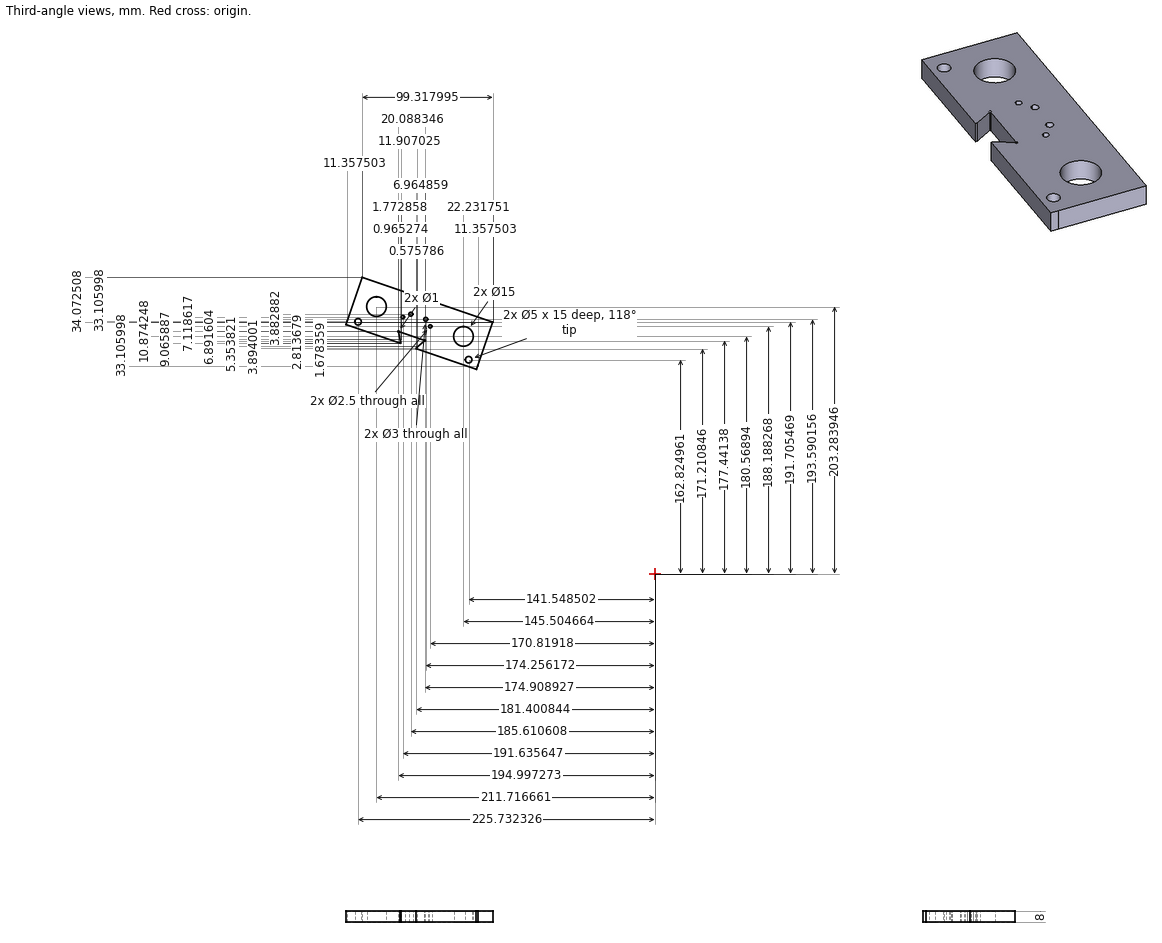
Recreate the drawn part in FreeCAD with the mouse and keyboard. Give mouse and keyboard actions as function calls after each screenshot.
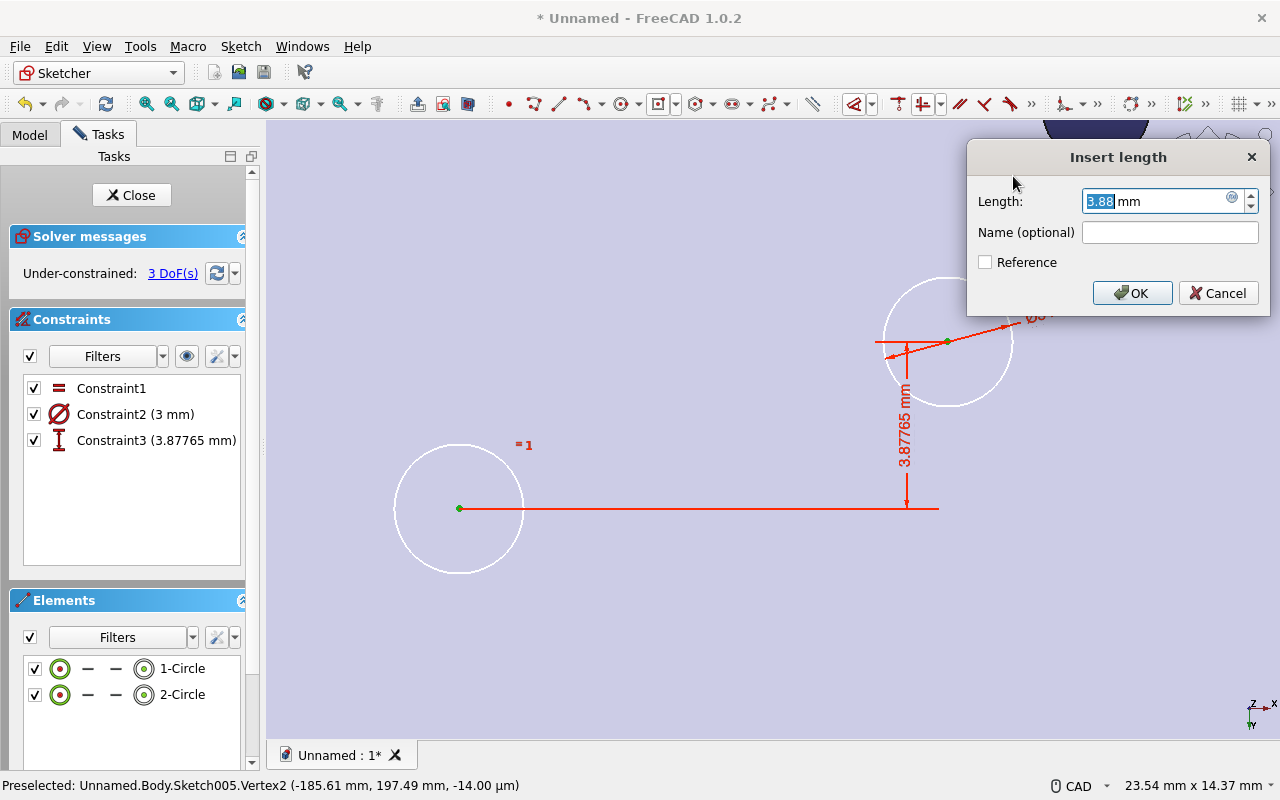
text(3.882882)
key(Return)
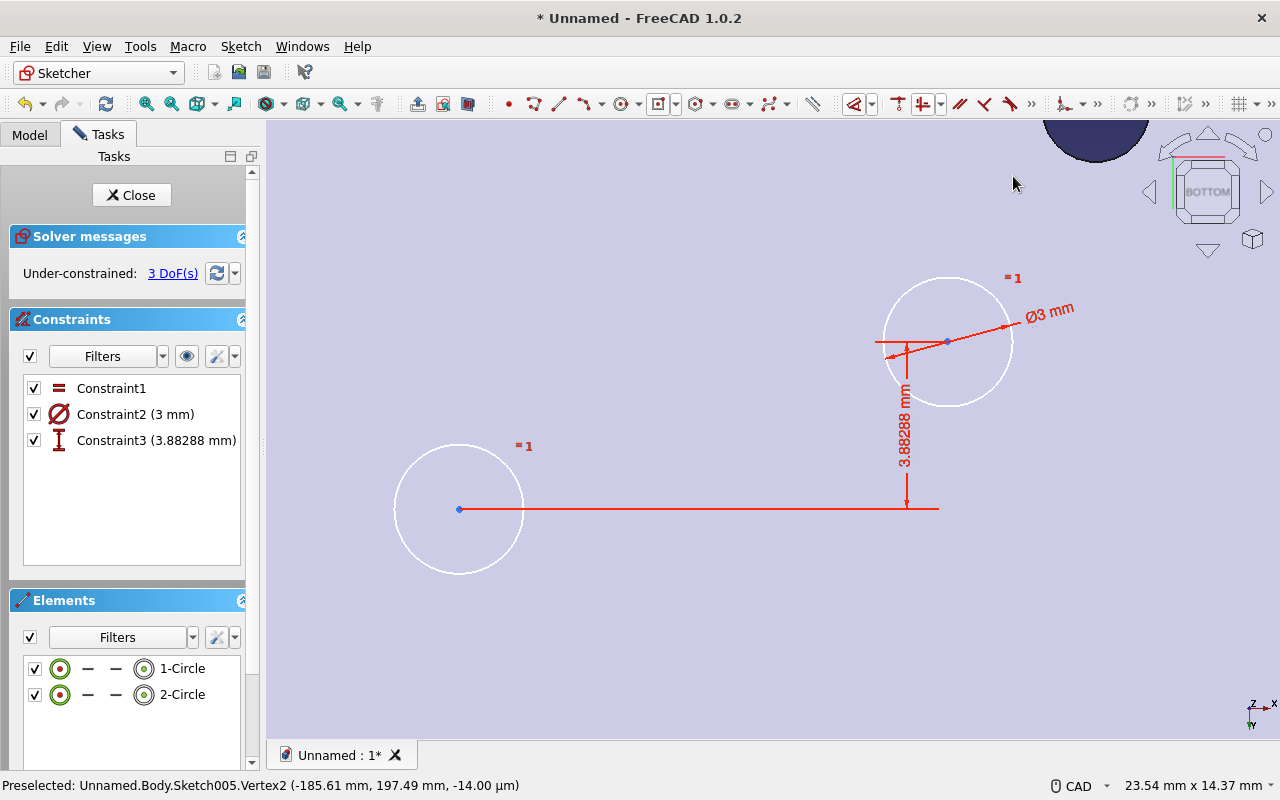
click(948, 342)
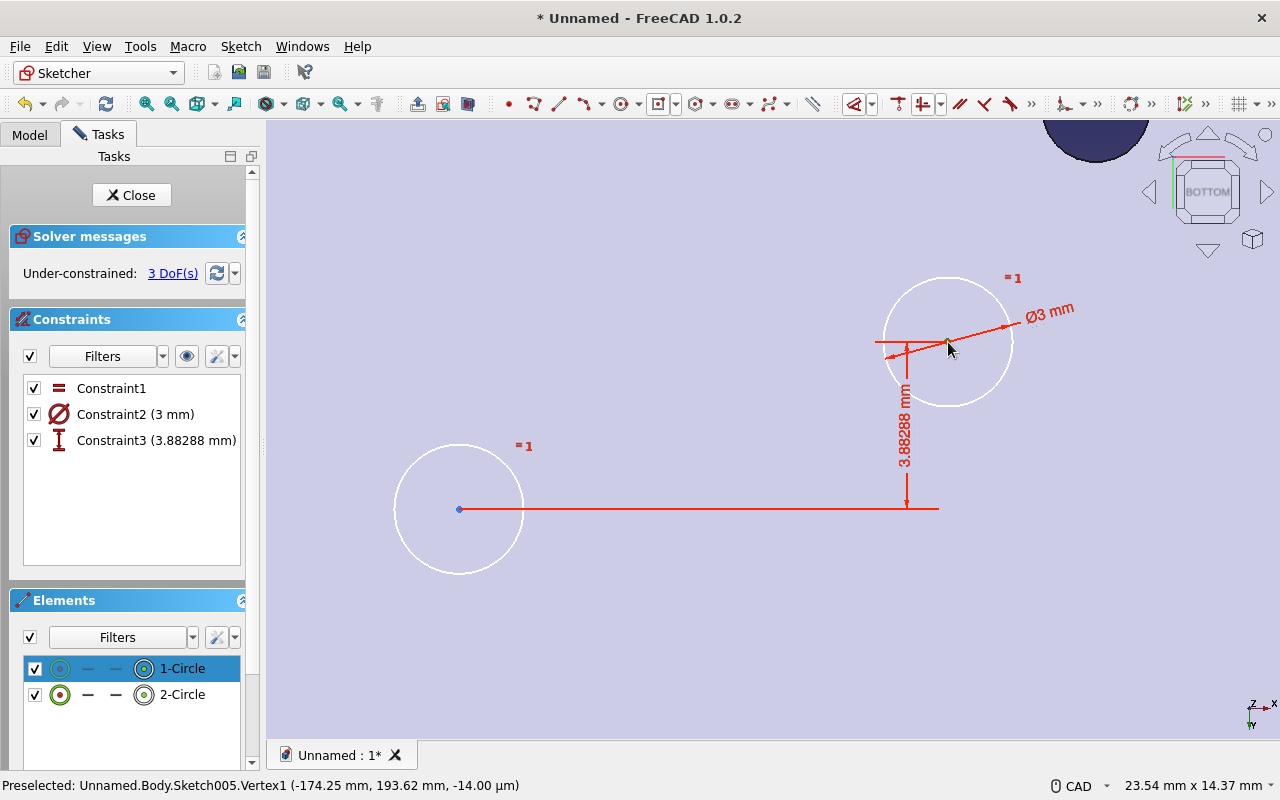
key(l)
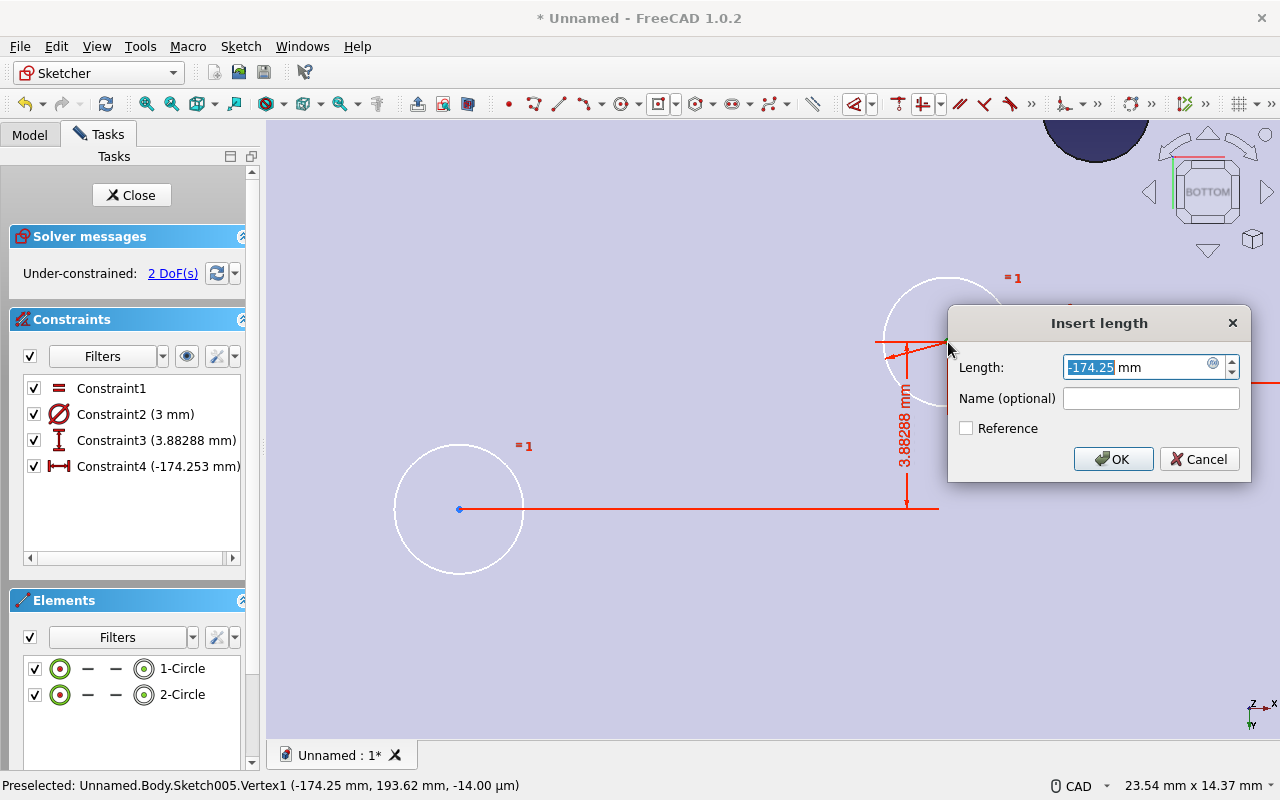
text(-174.256172)
key(Return)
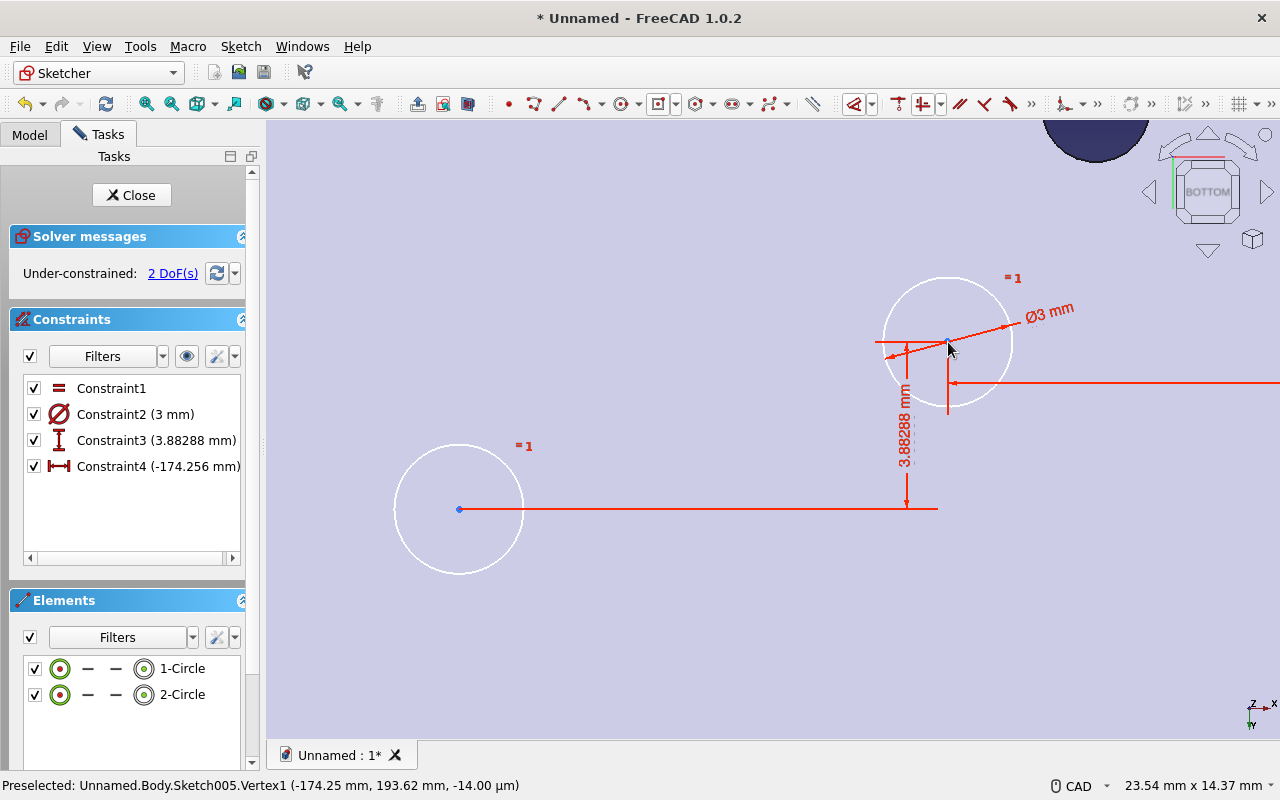
click(948, 342)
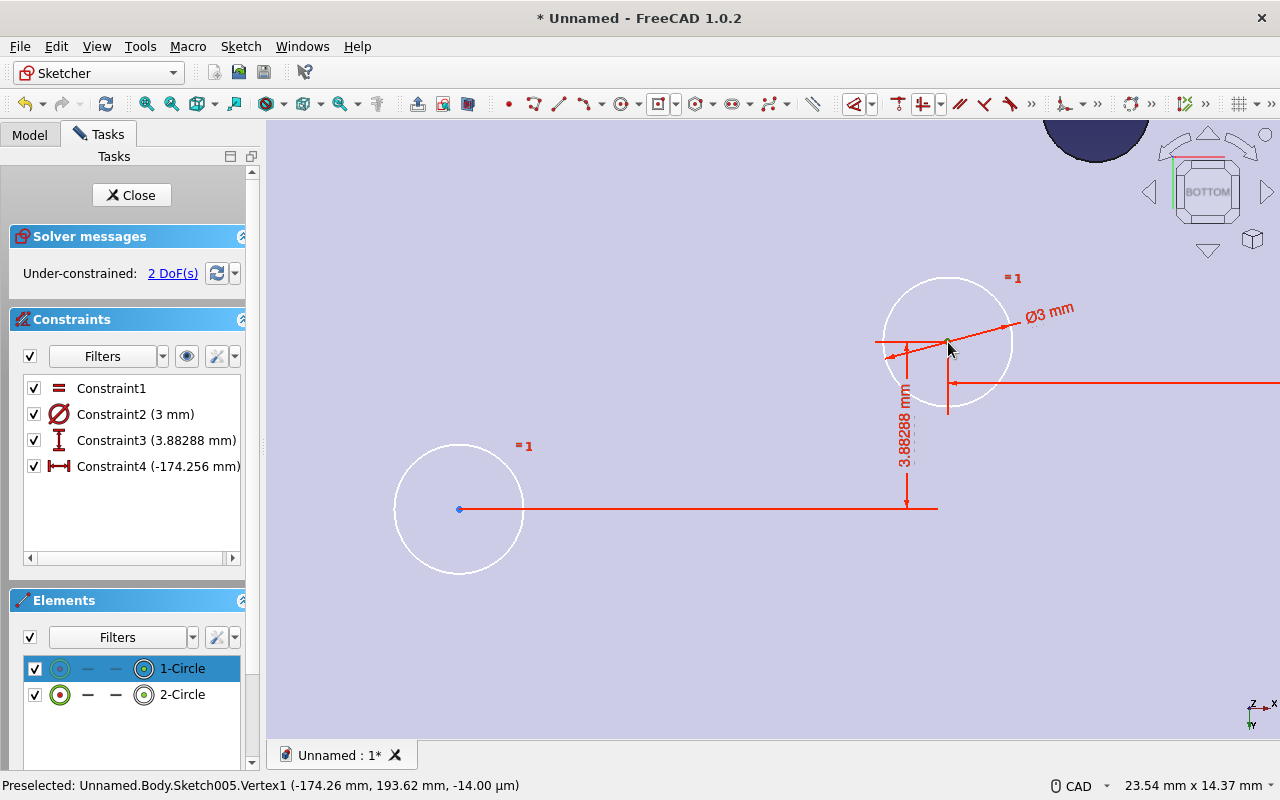
click(872, 104)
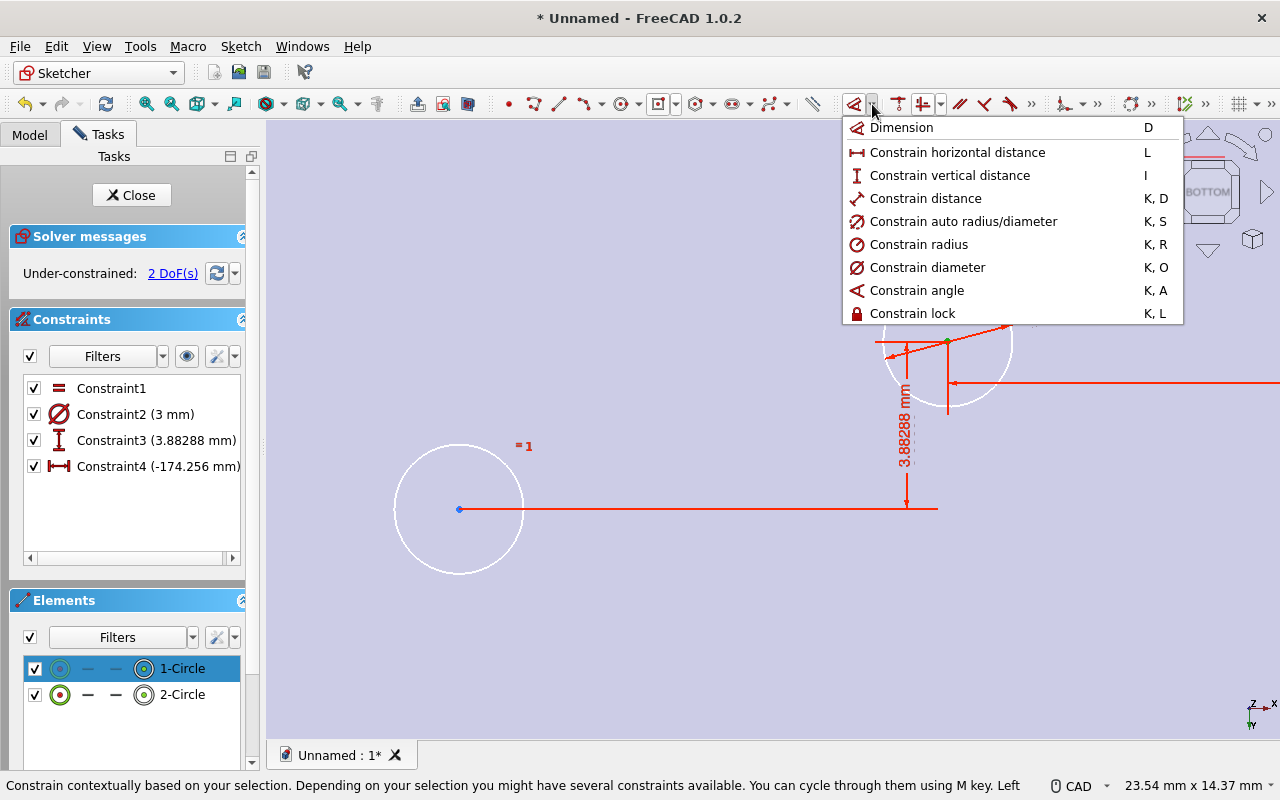
click(1013, 176)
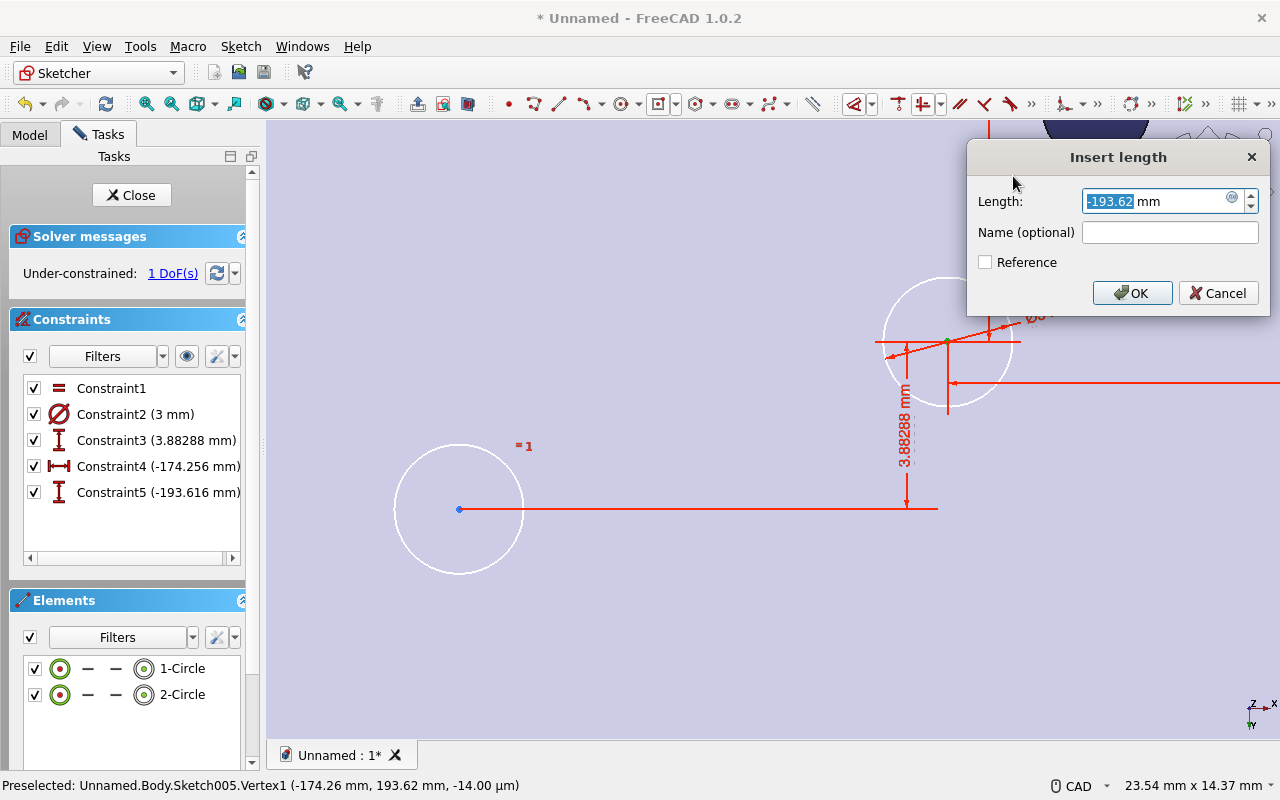
text(-193.590156)
key(Return)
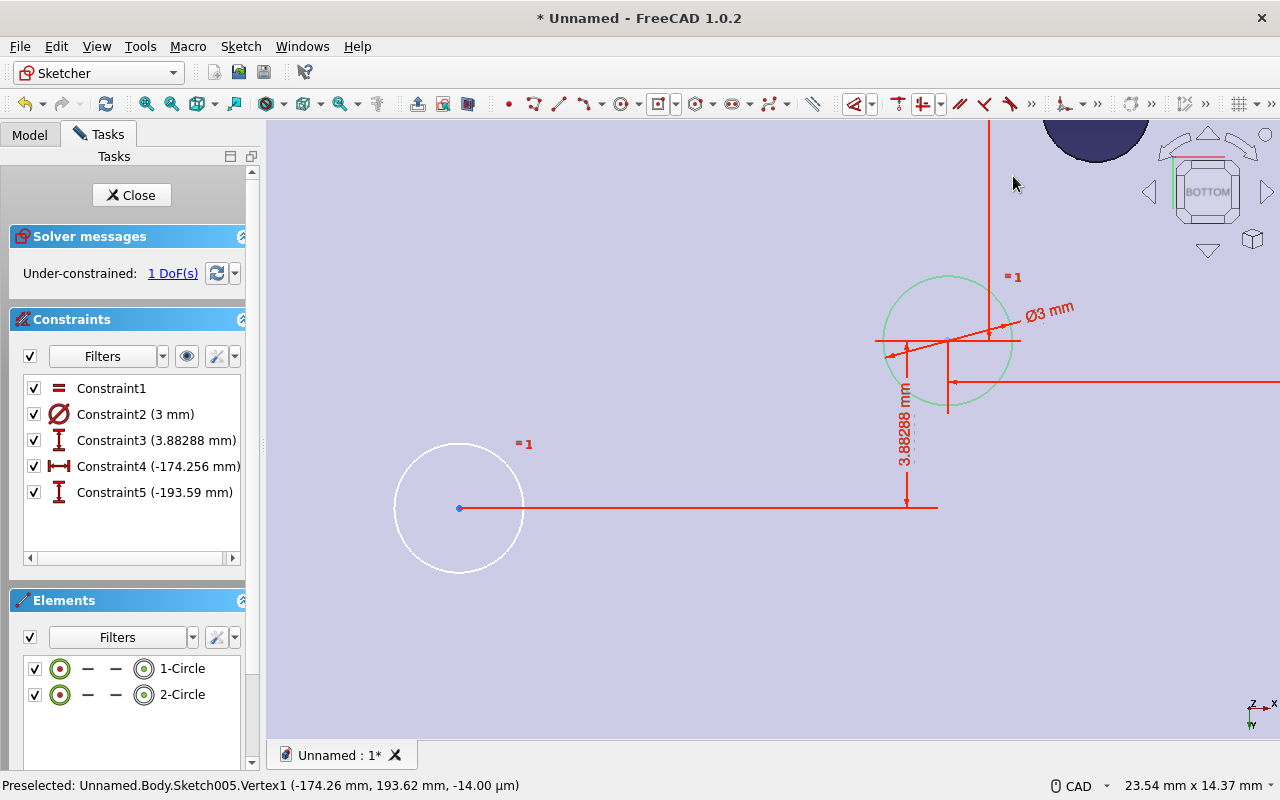
click(459, 508)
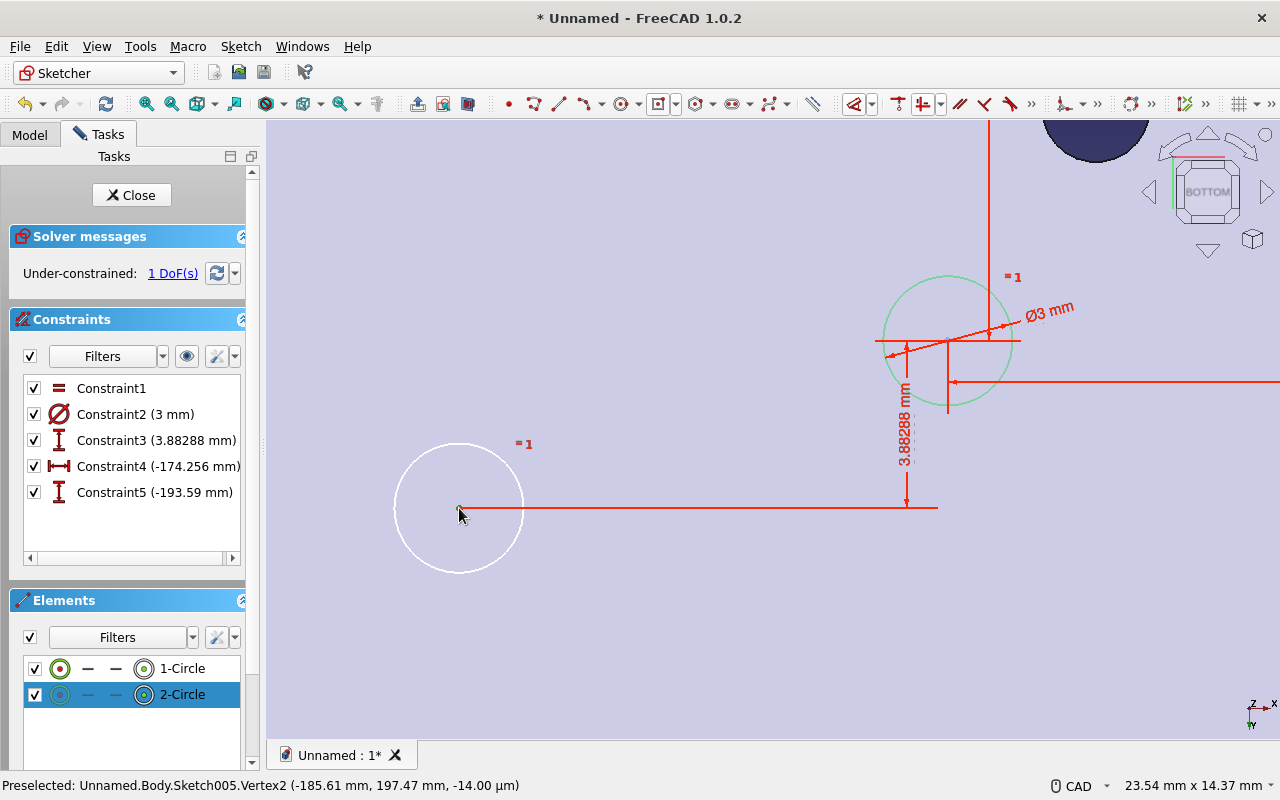
key(l)